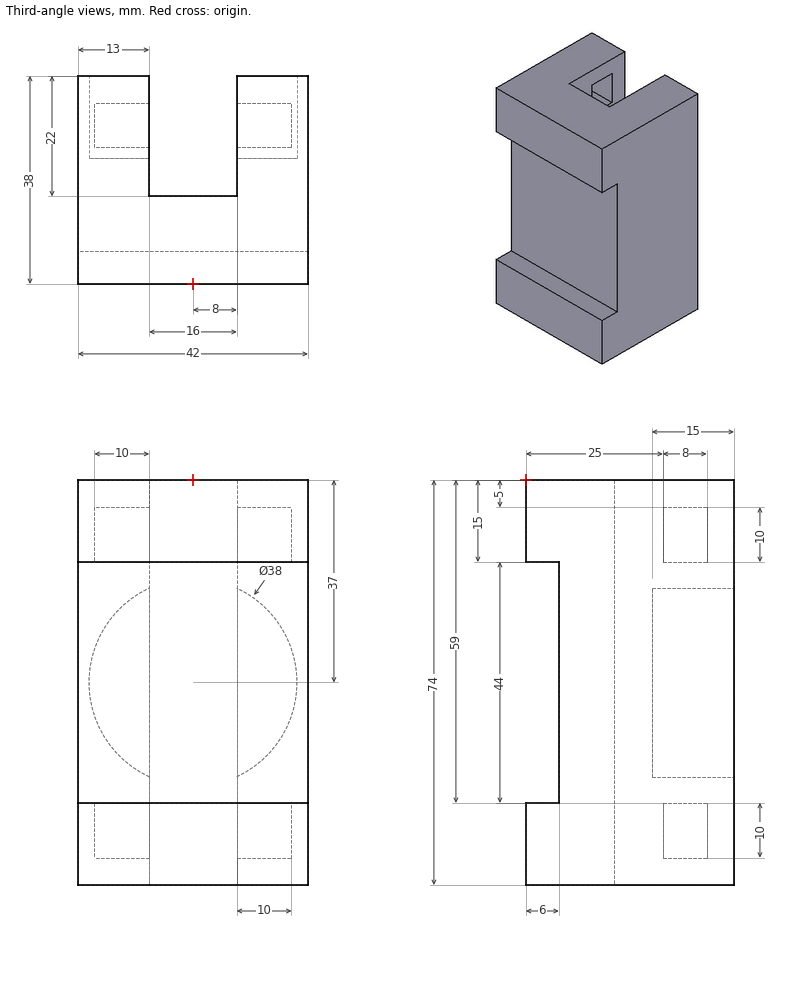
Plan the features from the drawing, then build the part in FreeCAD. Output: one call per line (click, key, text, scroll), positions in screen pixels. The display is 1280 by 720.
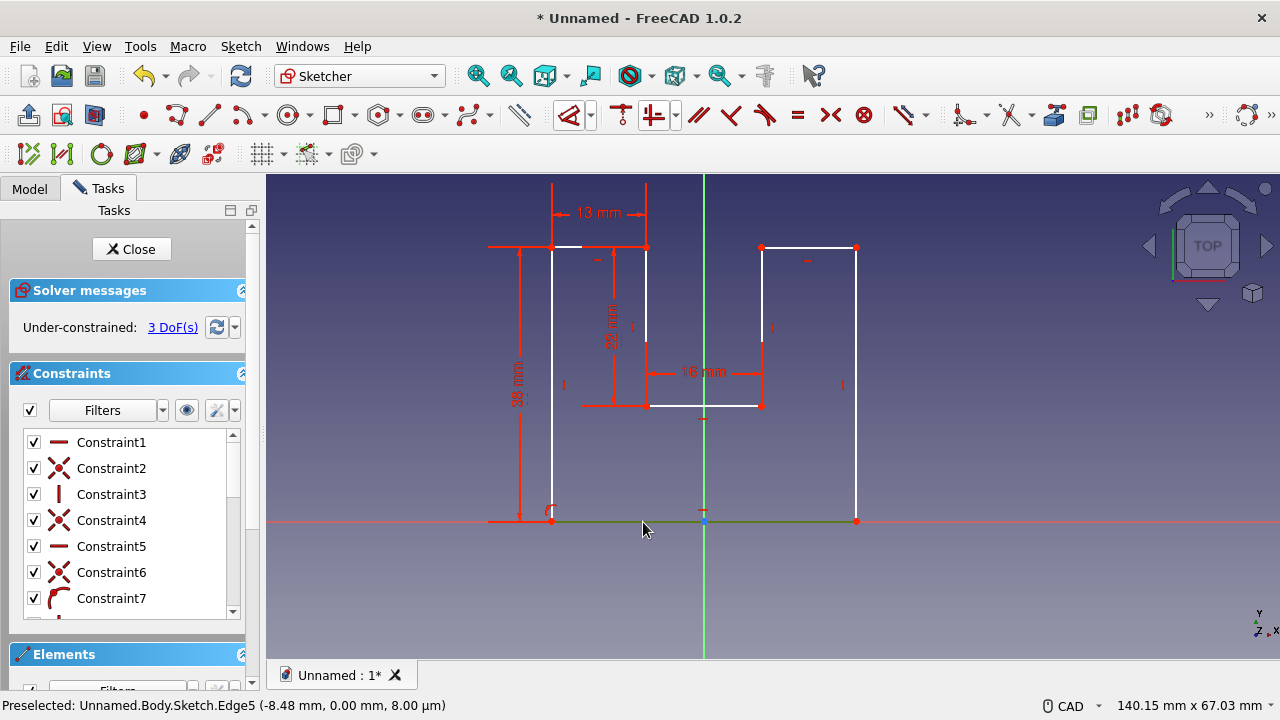
click(590, 116)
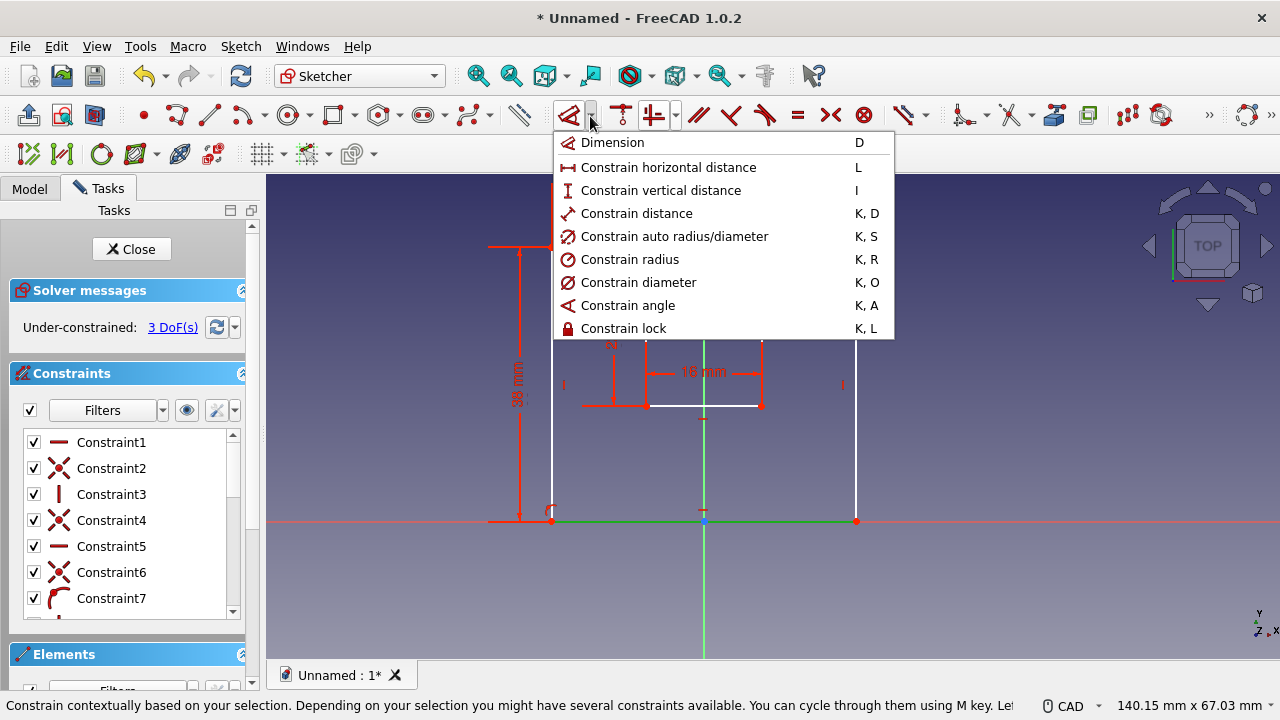
click(724, 168)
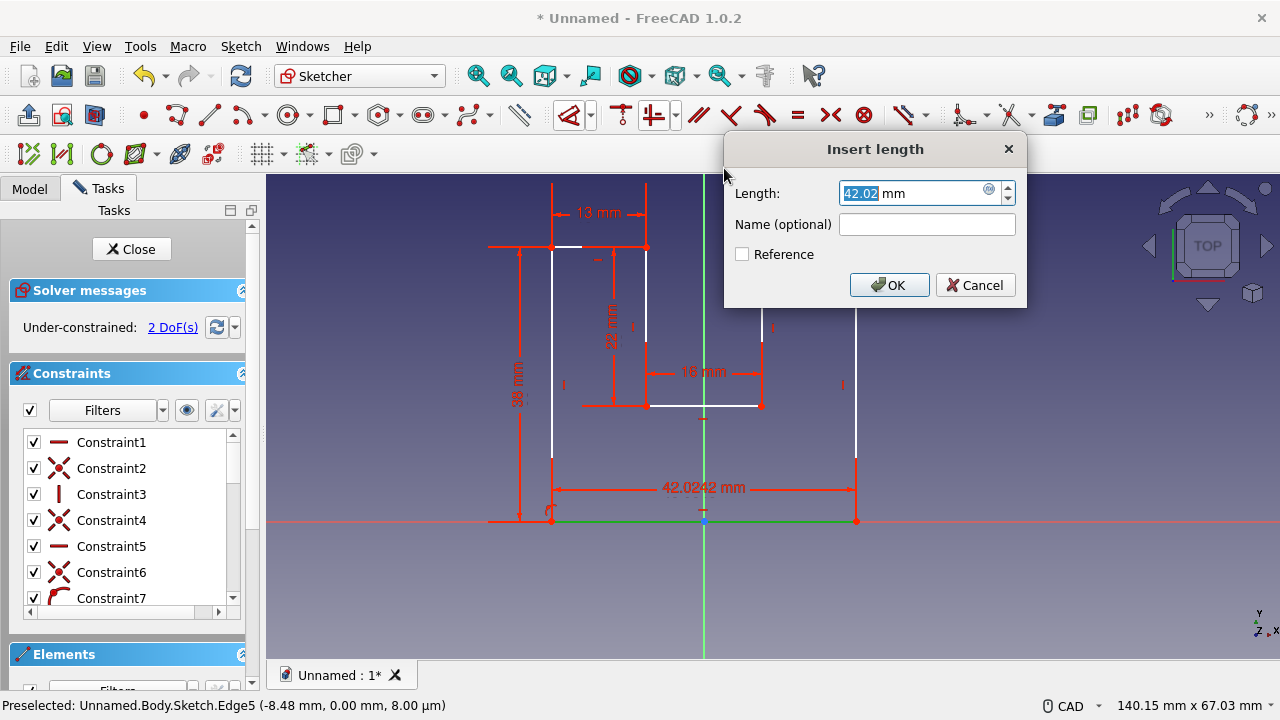
text(42)
key(Return)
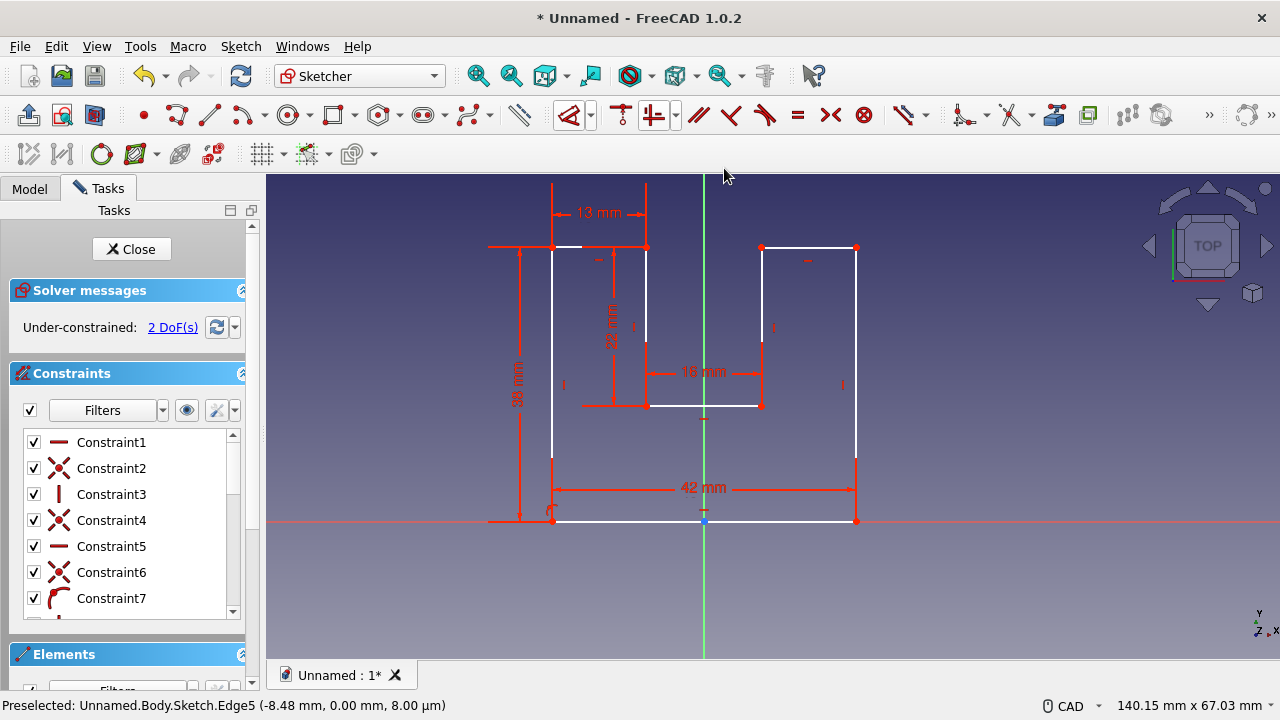
click(856, 440)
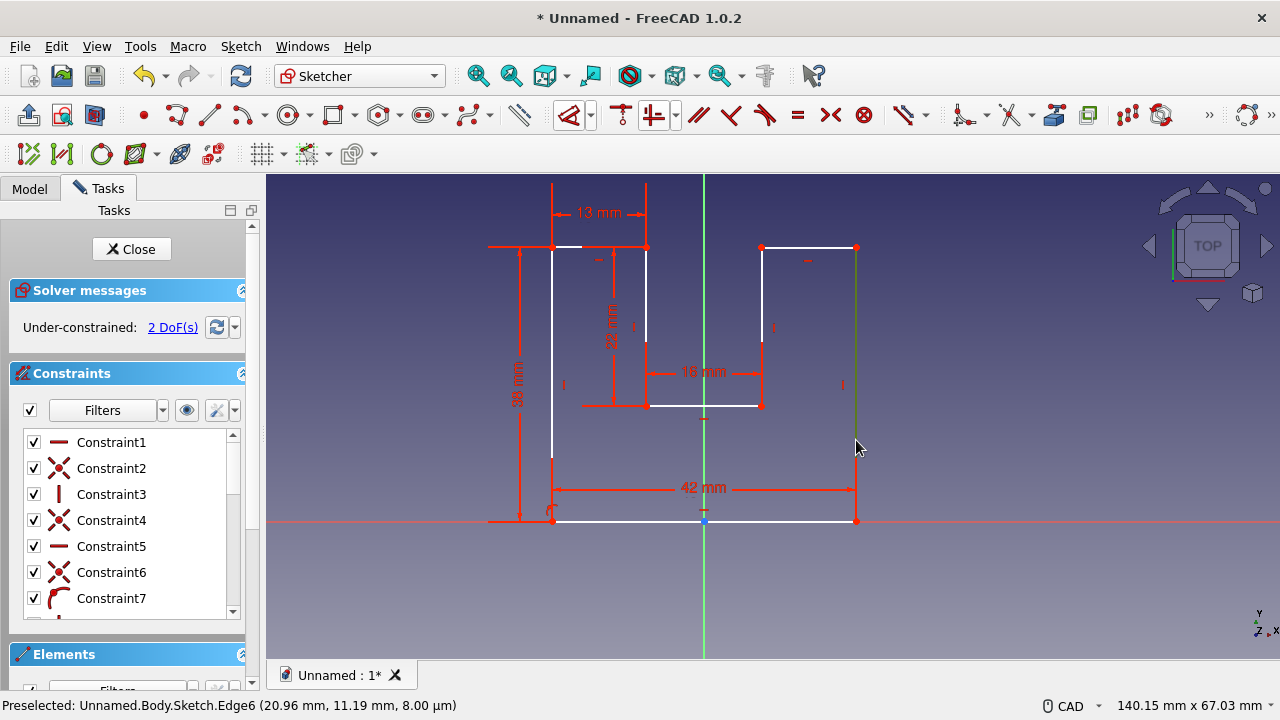
key(i)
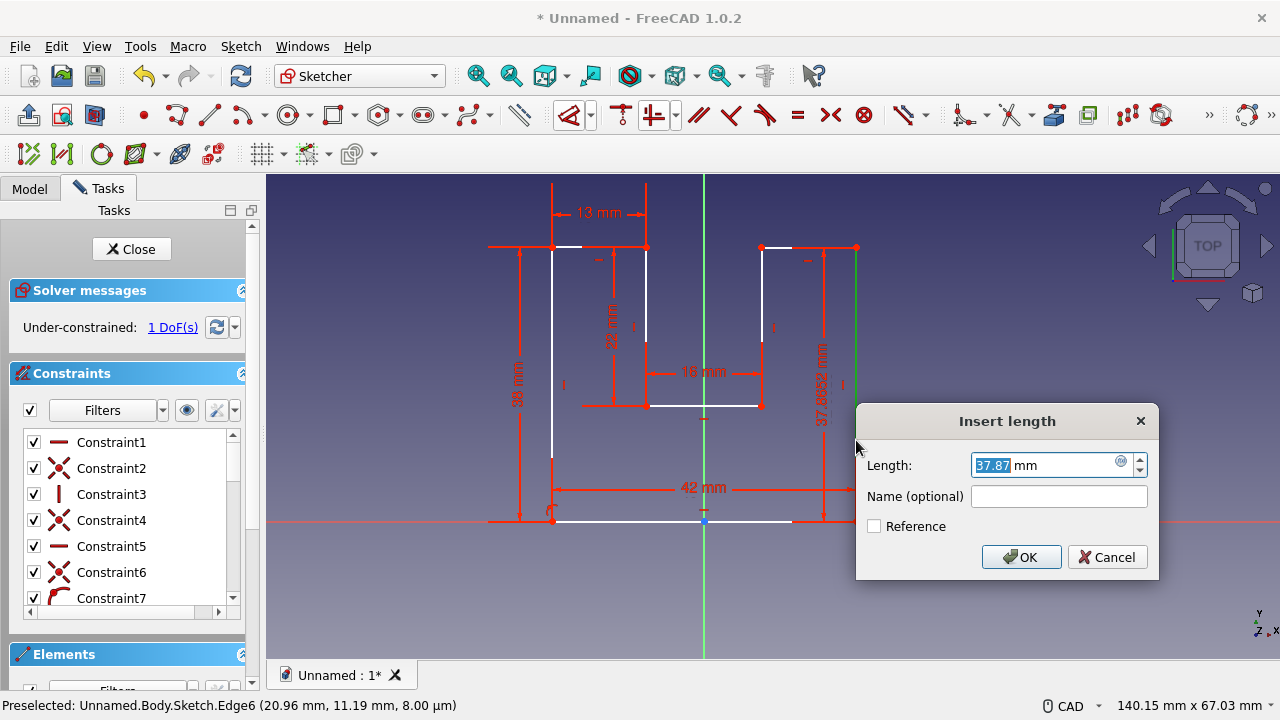
text(38)
key(Return)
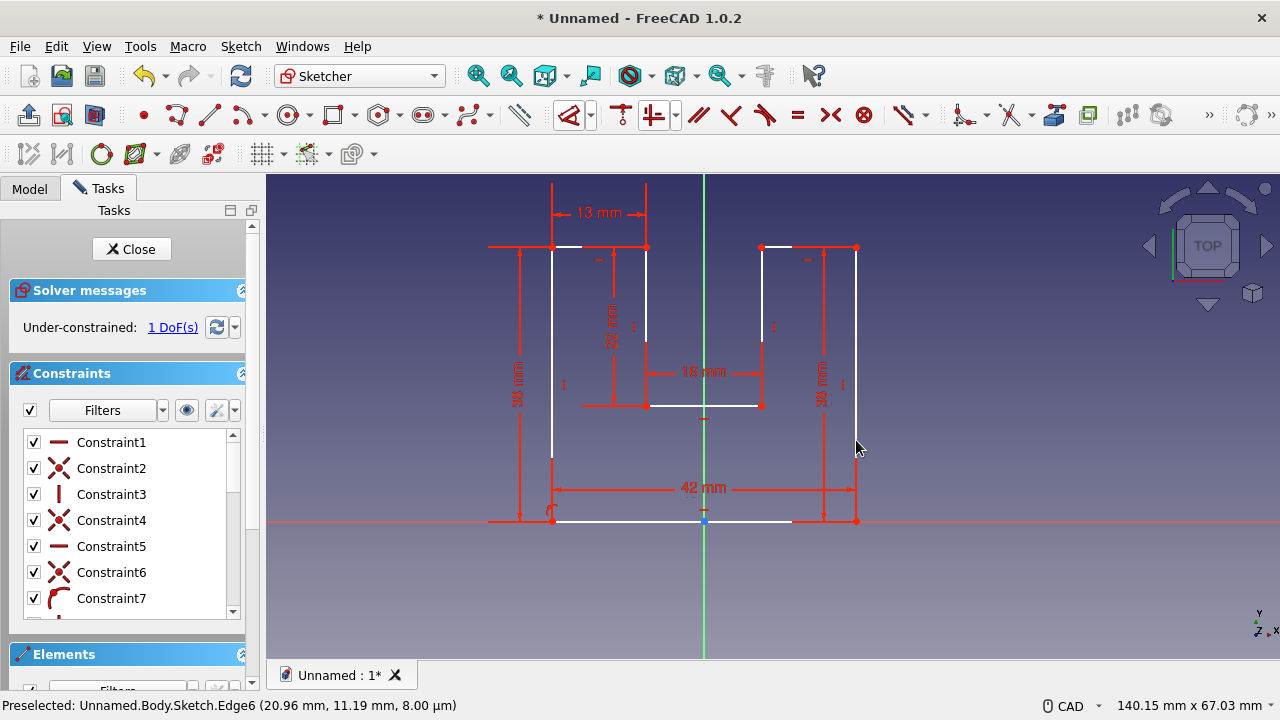
click(762, 406)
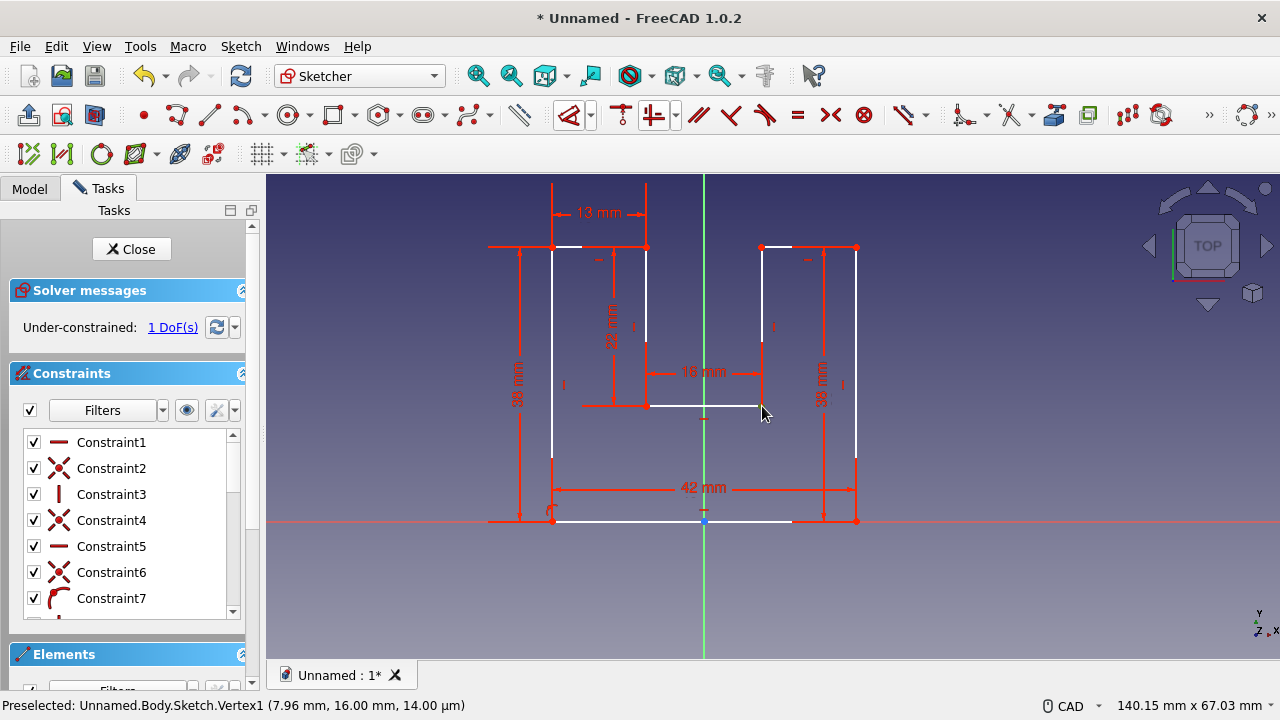
key(l)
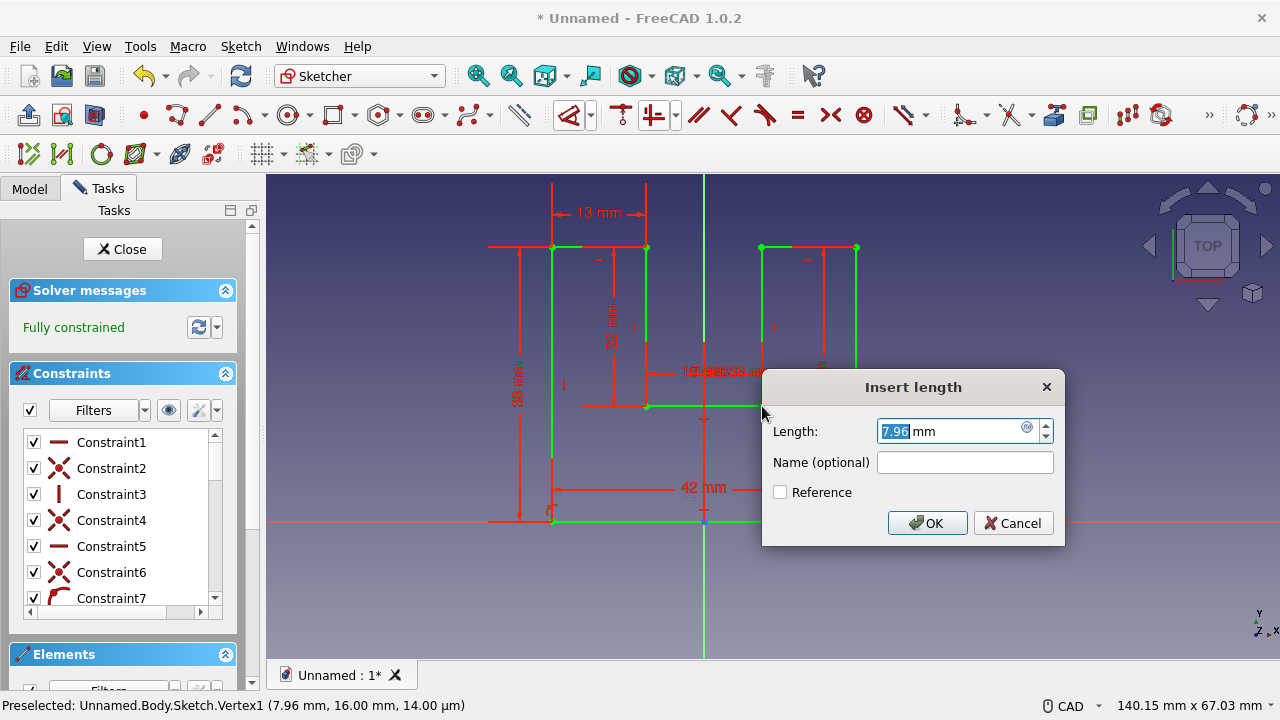
text(8)
key(Return)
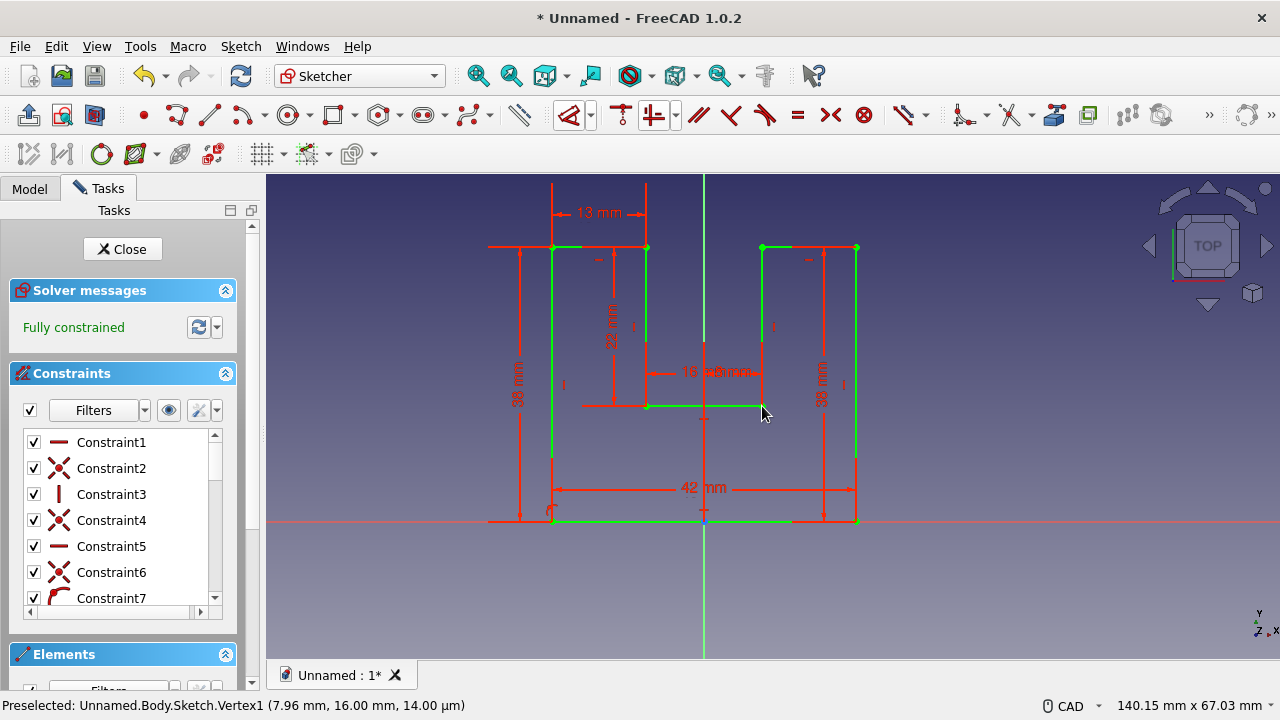
click(123, 249)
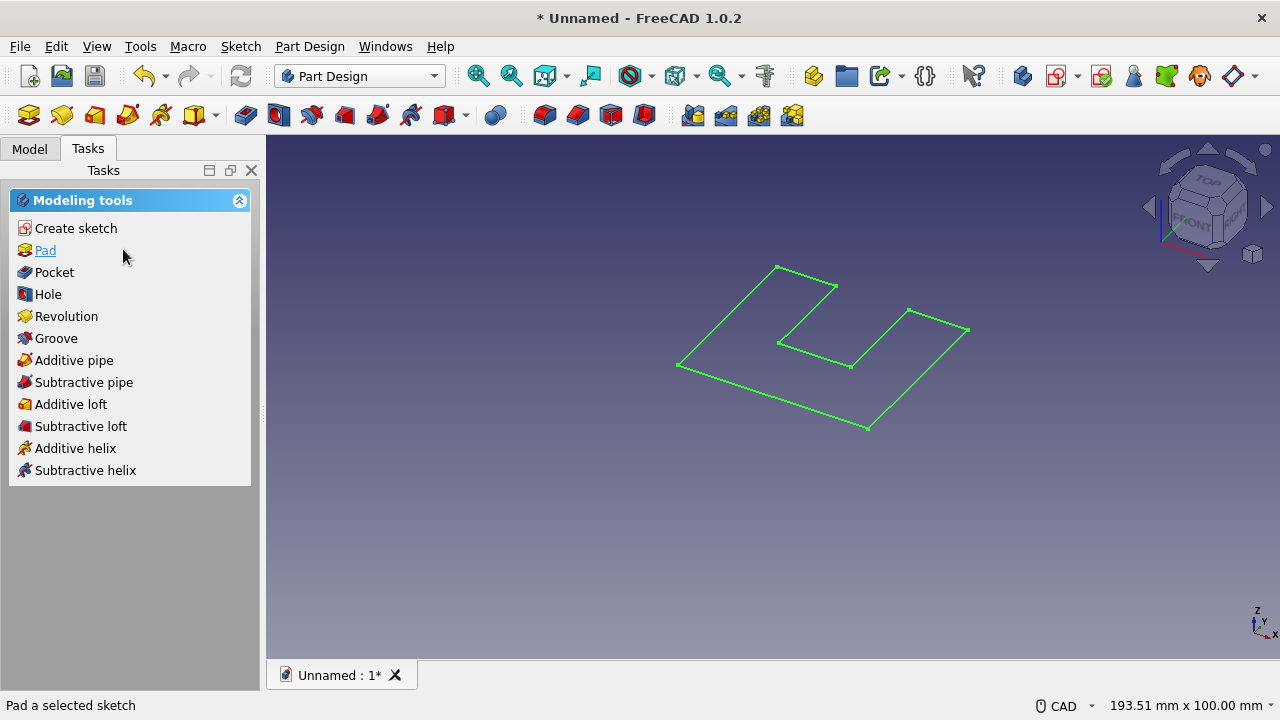
click(29, 116)